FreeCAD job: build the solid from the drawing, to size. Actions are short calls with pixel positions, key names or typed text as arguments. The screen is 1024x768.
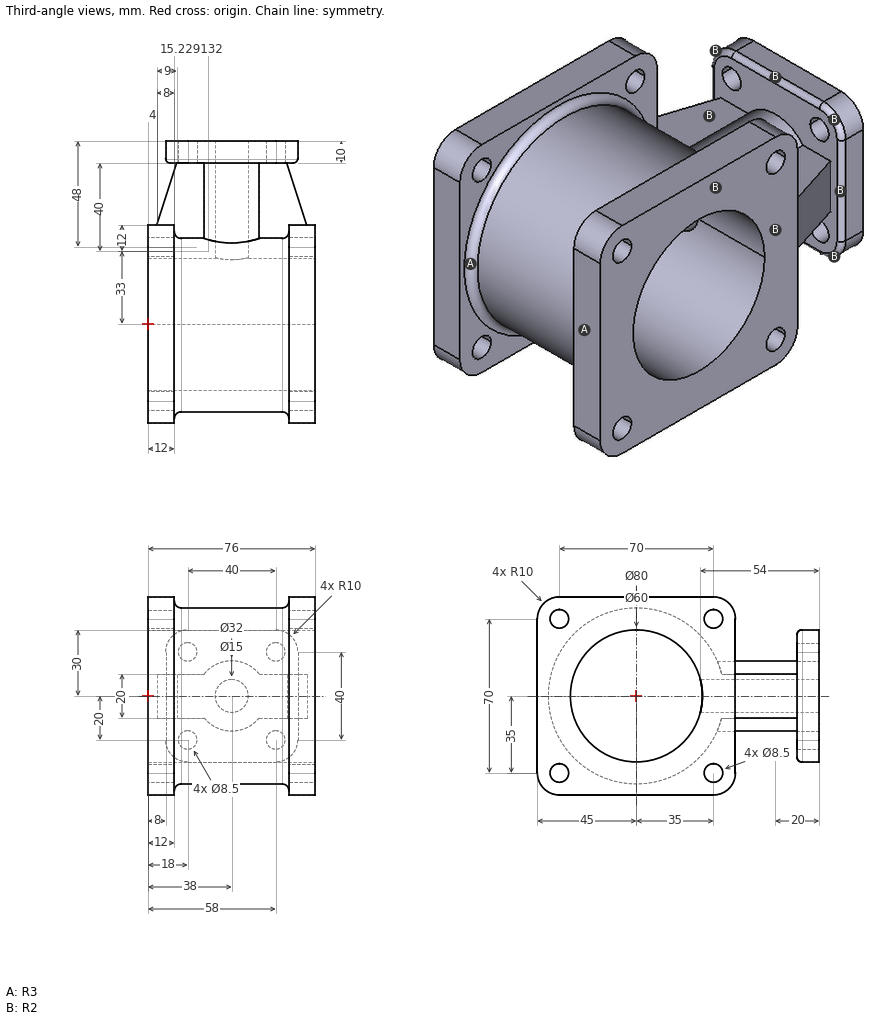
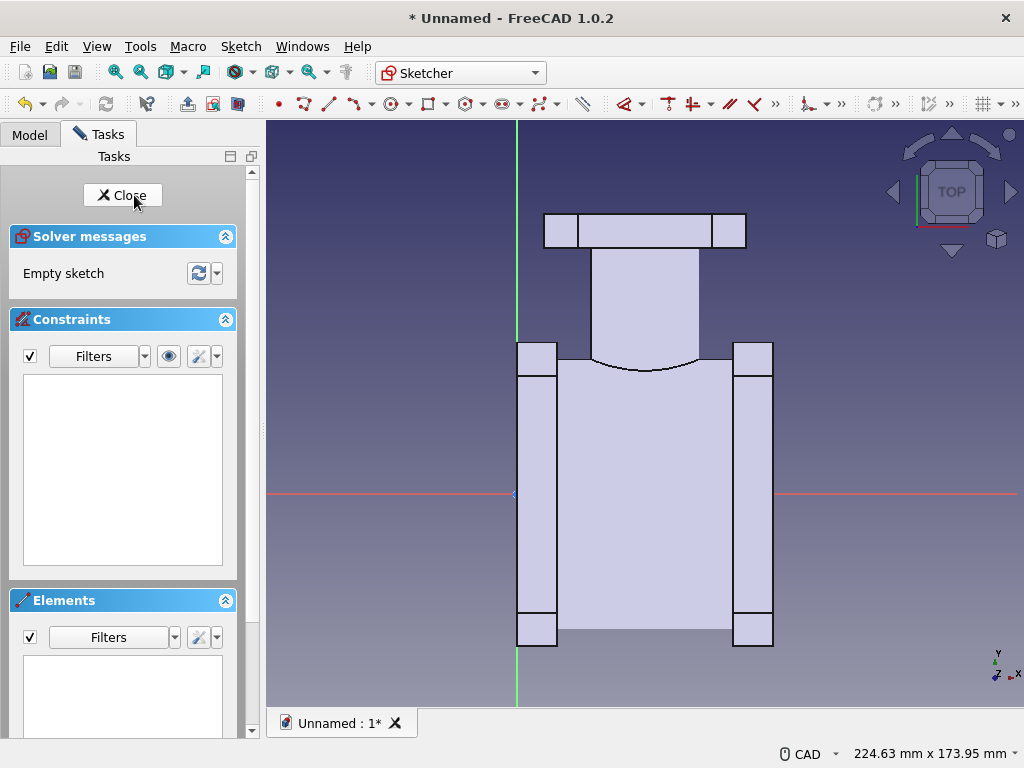
key(q)
key(s)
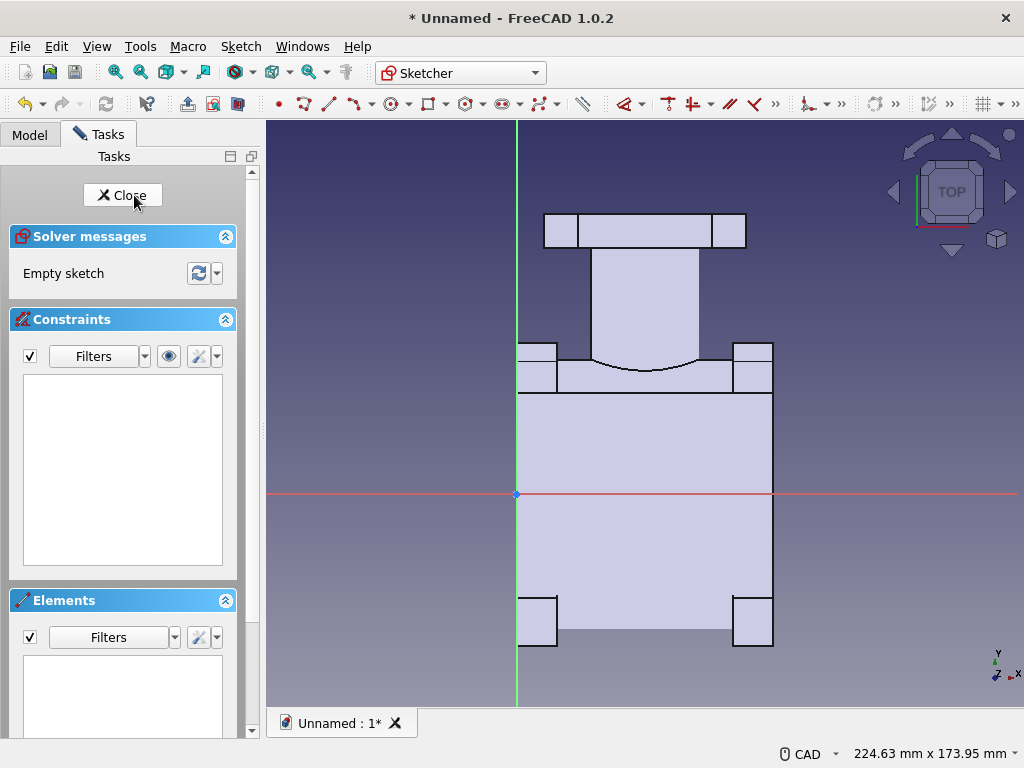
scroll(535, 286, up, 2)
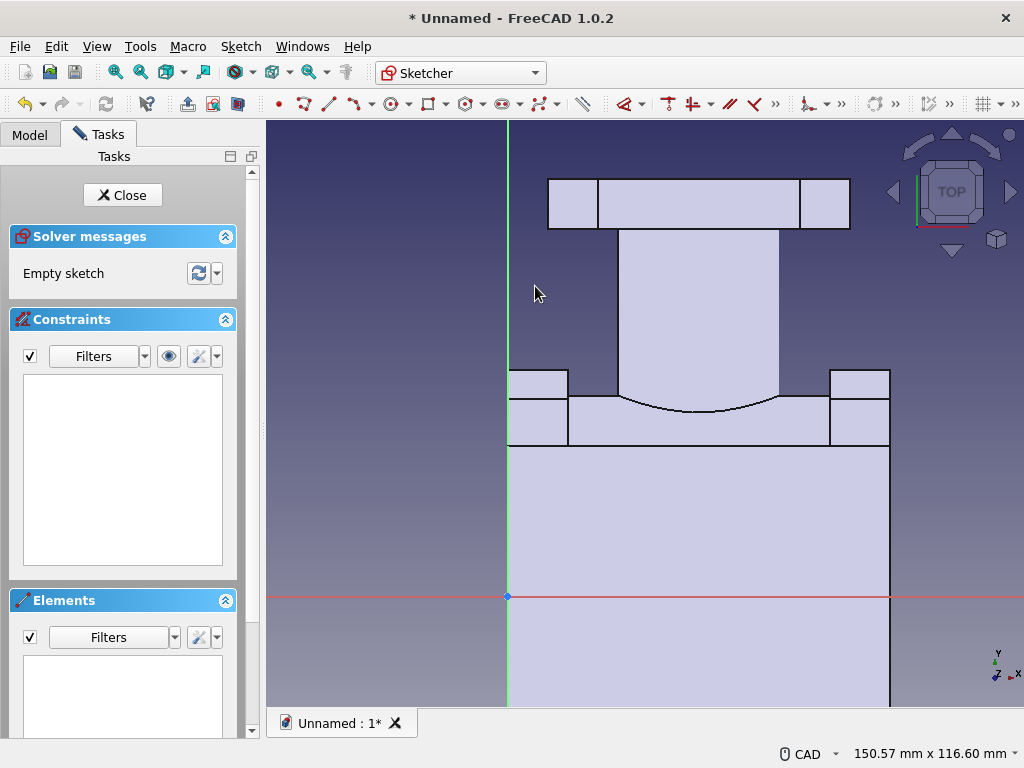
key(g)
key(m)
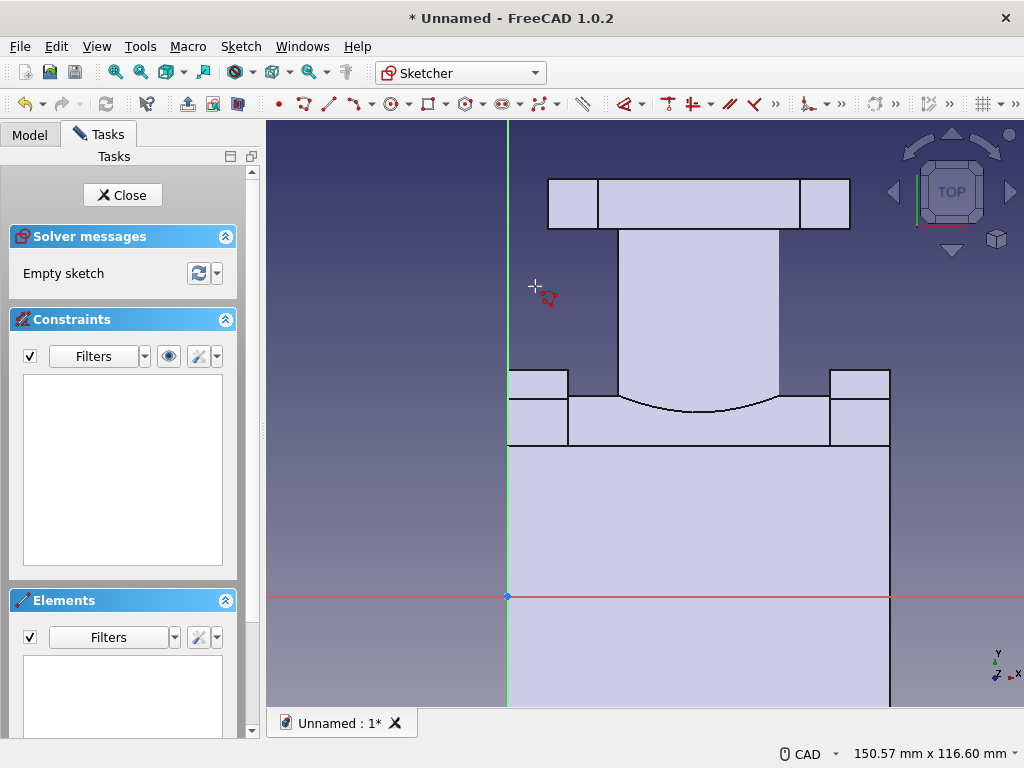
click(568, 431)
click(645, 431)
click(645, 229)
click(573, 229)
click(528, 370)
click(568, 370)
click(568, 432)
key(Escape)
key(Escape)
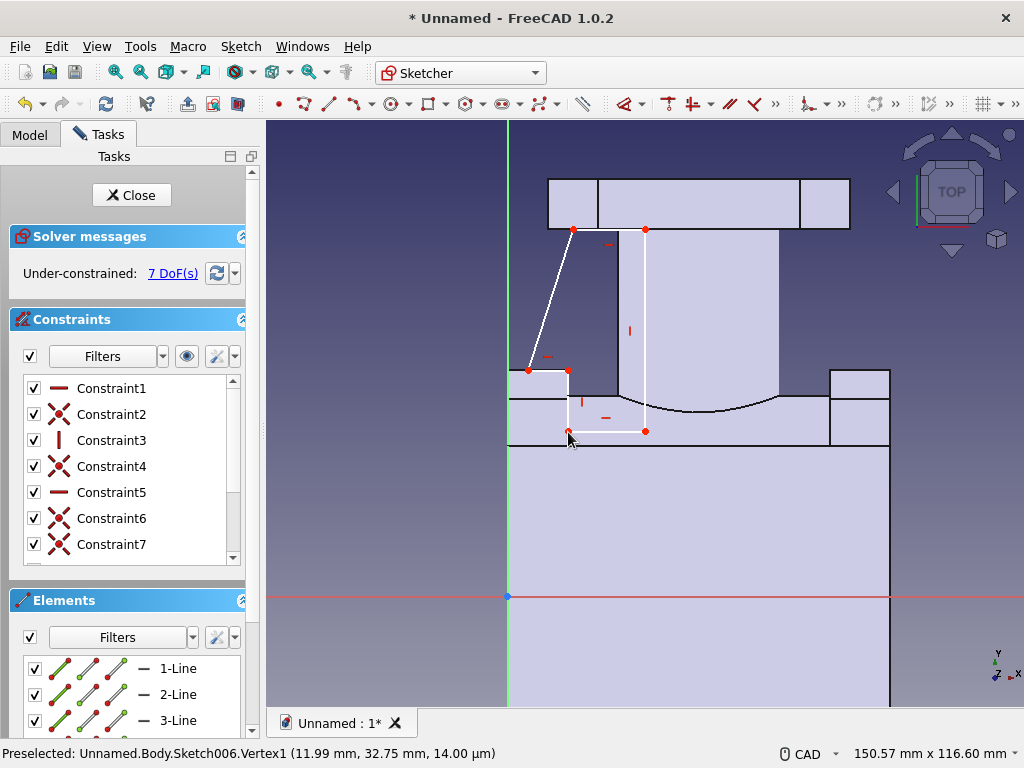
key(d)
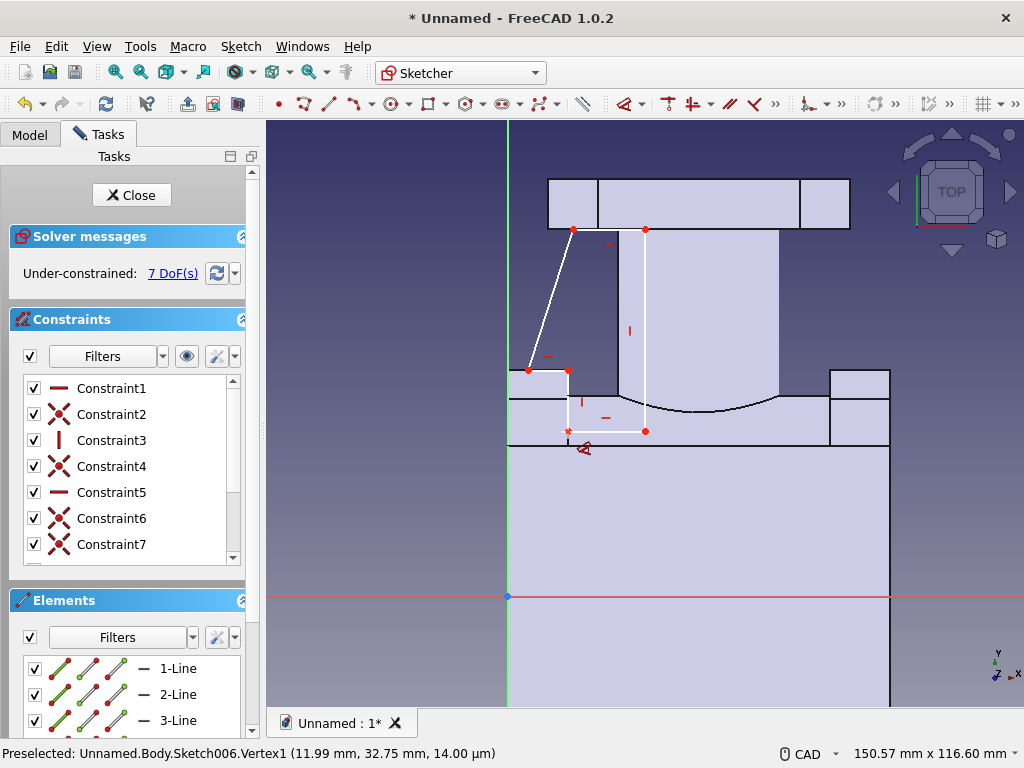
click(540, 371)
click(557, 337)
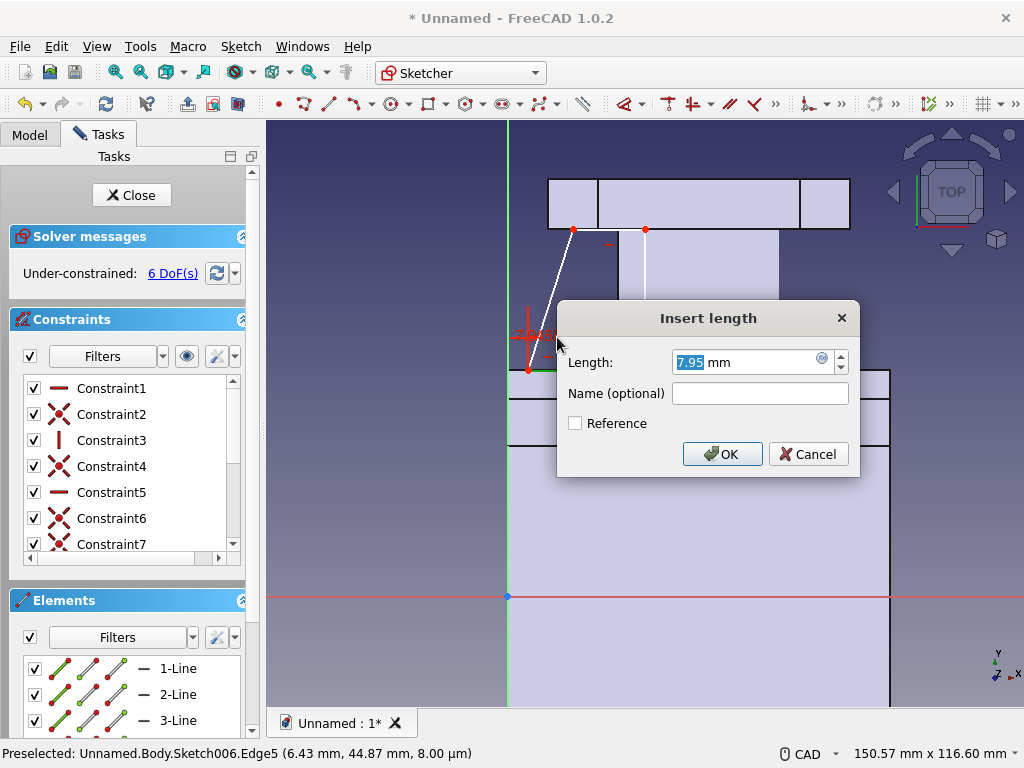
text(8)
key(Return)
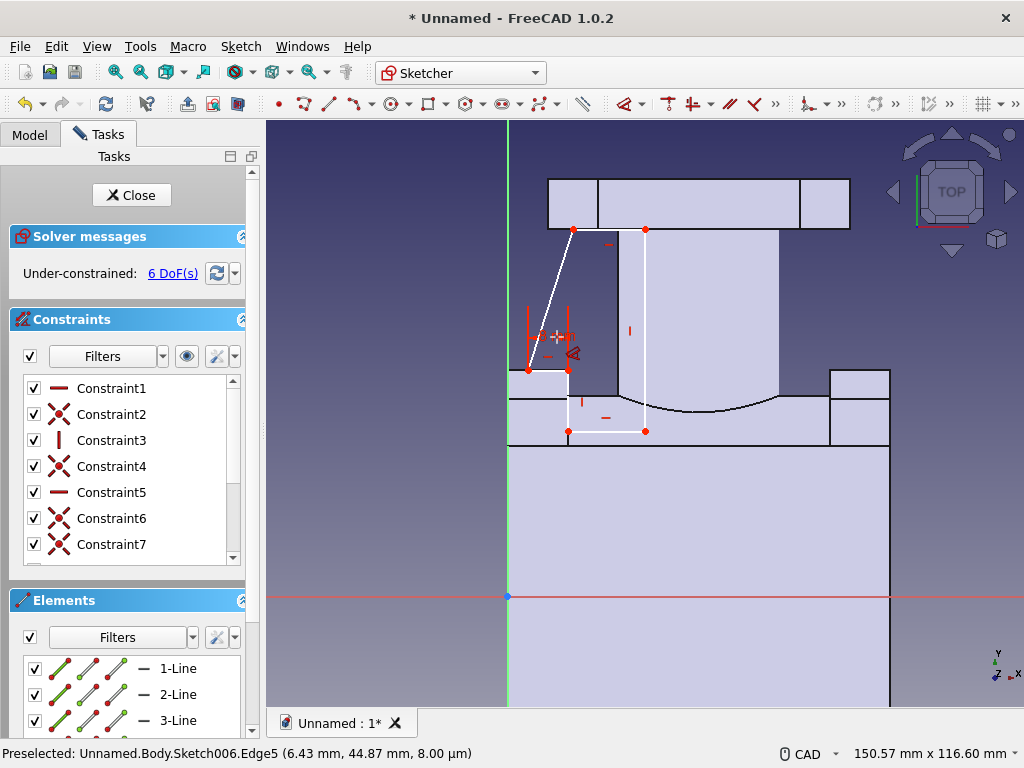
click(645, 371)
click(679, 331)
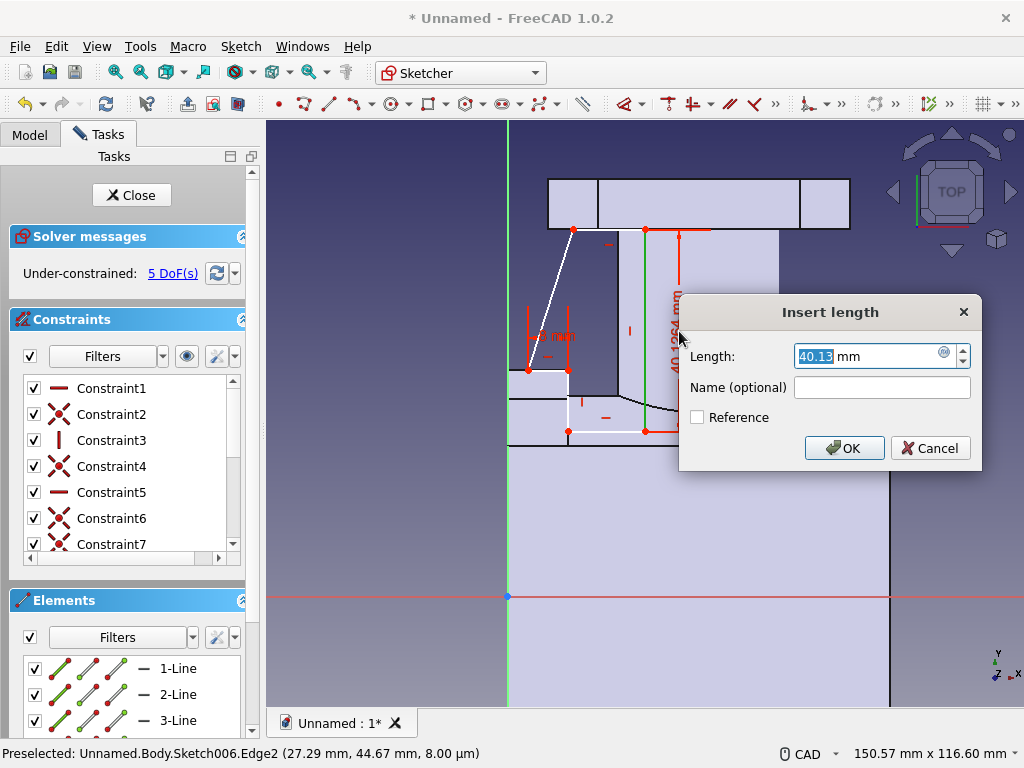
text(40)
key(Return)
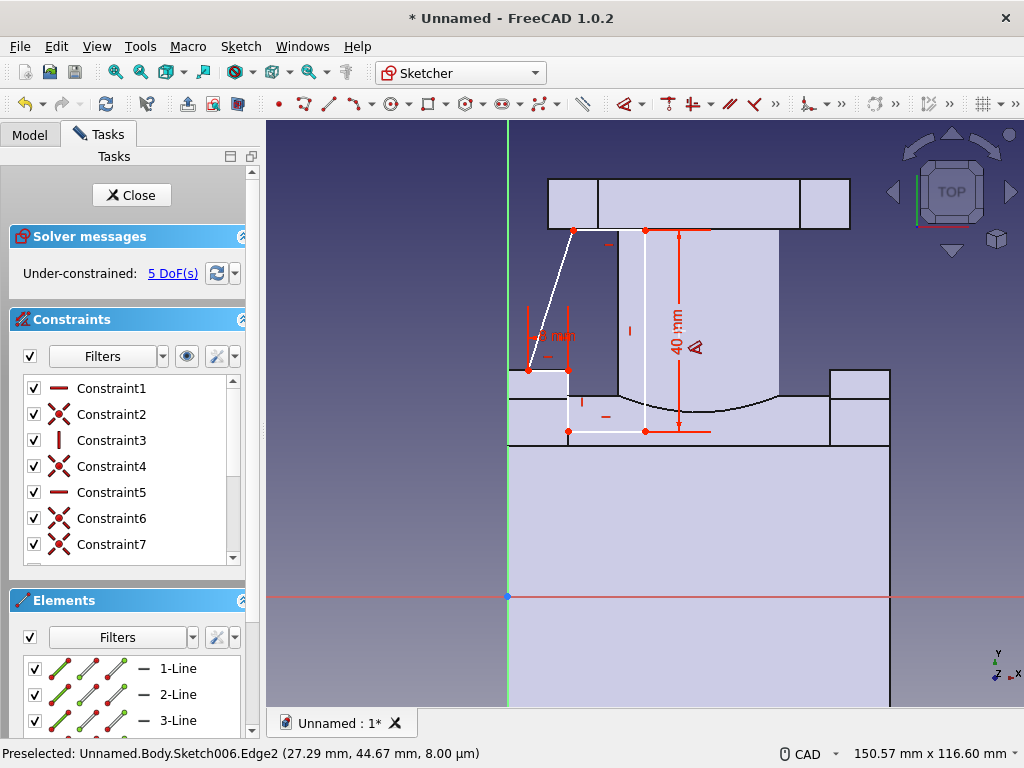
click(568, 389)
click(534, 401)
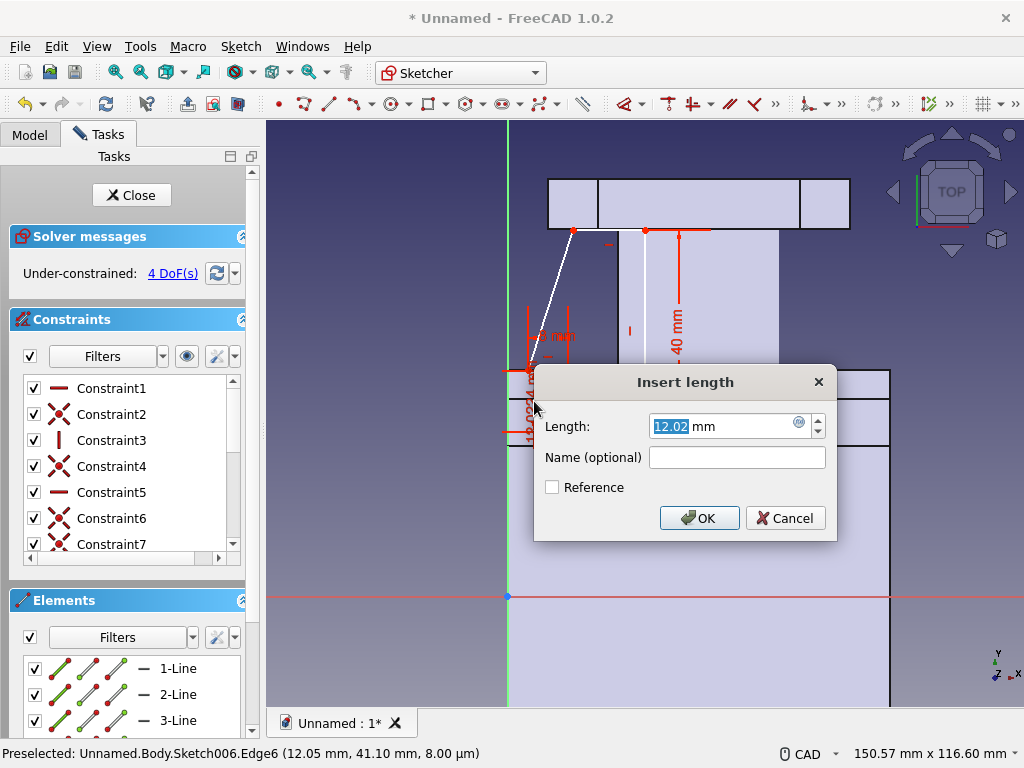
text(12)
key(Return)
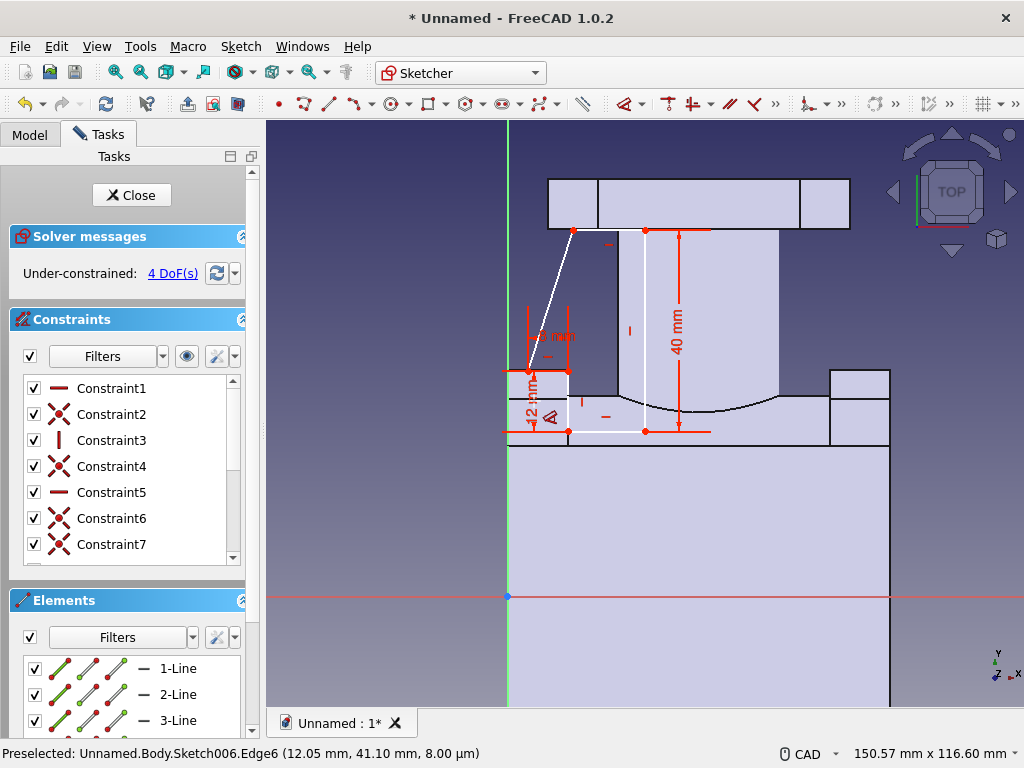
scroll(528, 371, up, 4)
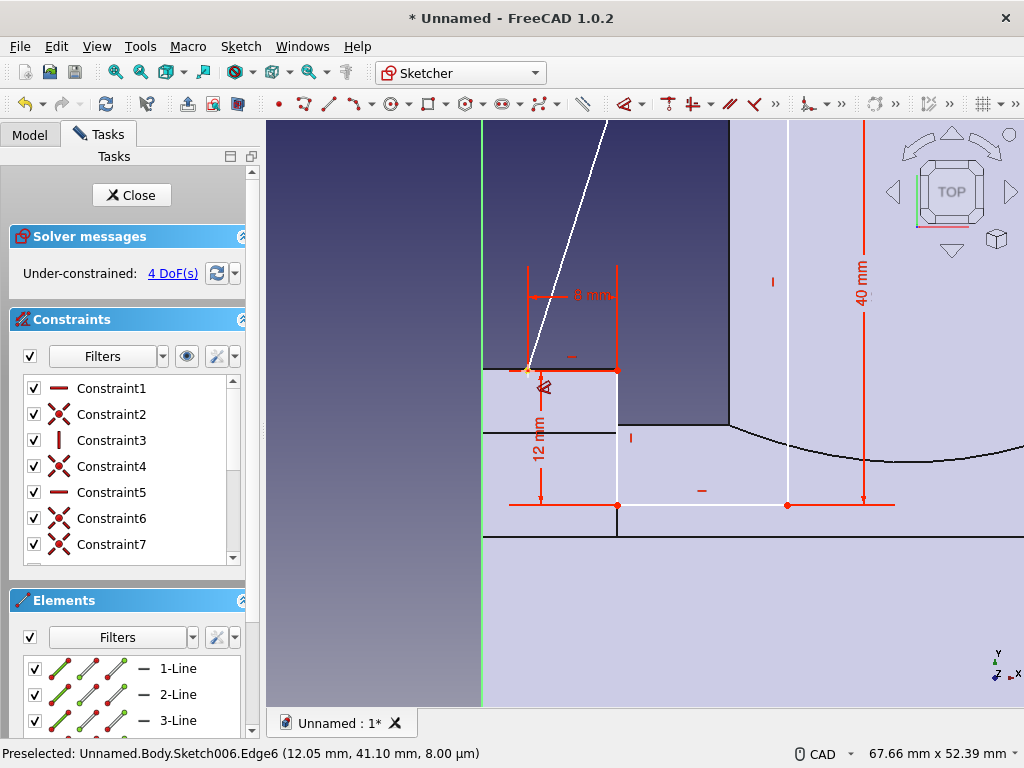
click(528, 371)
click(505, 337)